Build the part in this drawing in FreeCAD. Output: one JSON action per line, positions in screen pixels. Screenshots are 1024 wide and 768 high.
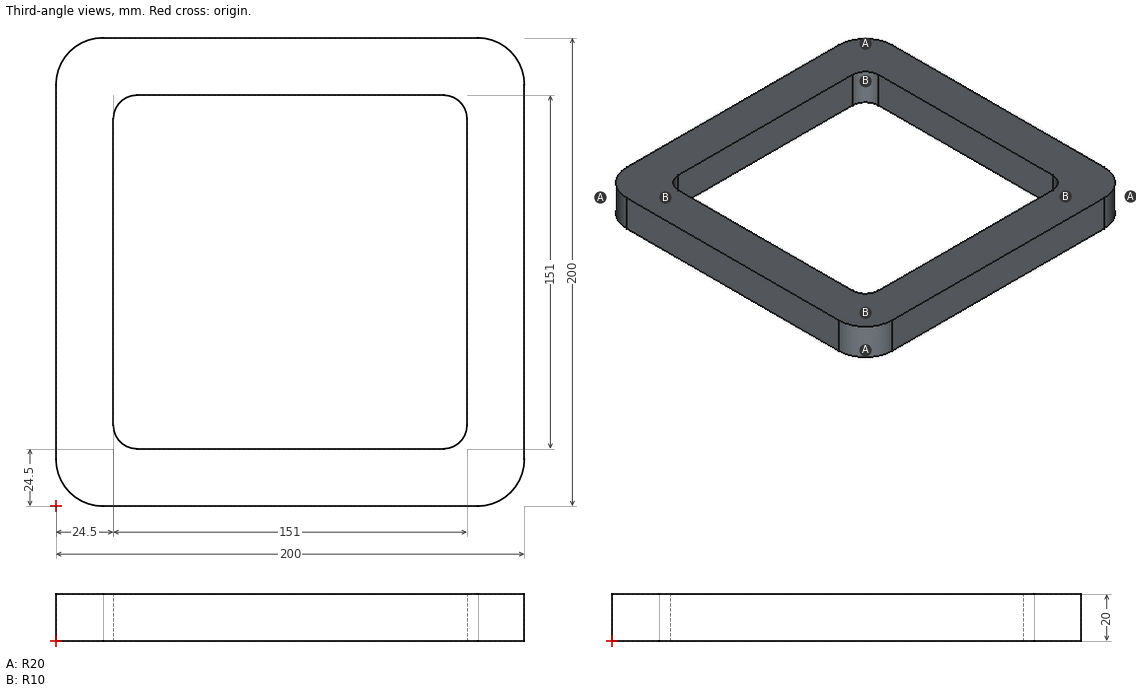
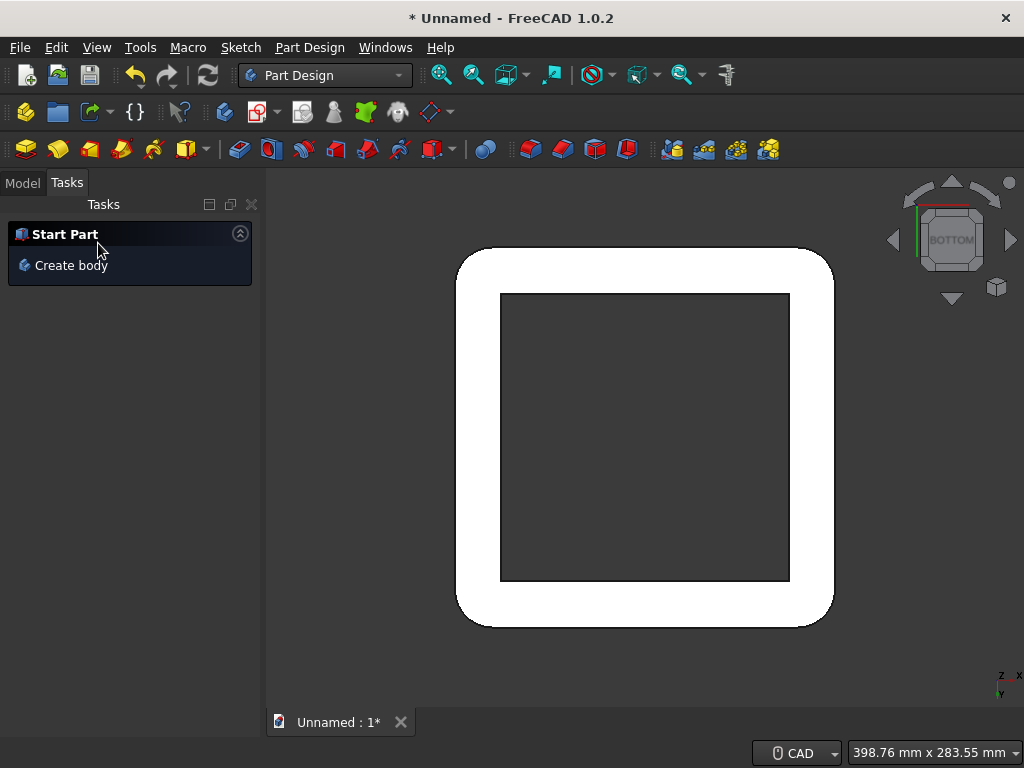
{"action": "key", "text": "4"}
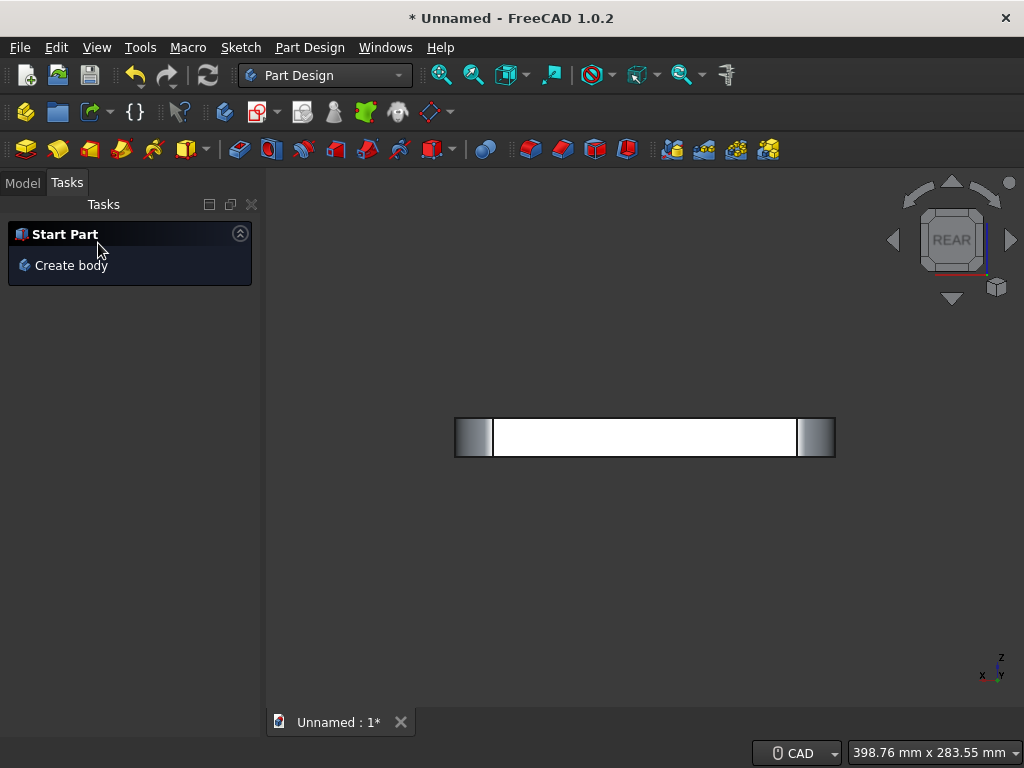
{"action": "key", "text": "6"}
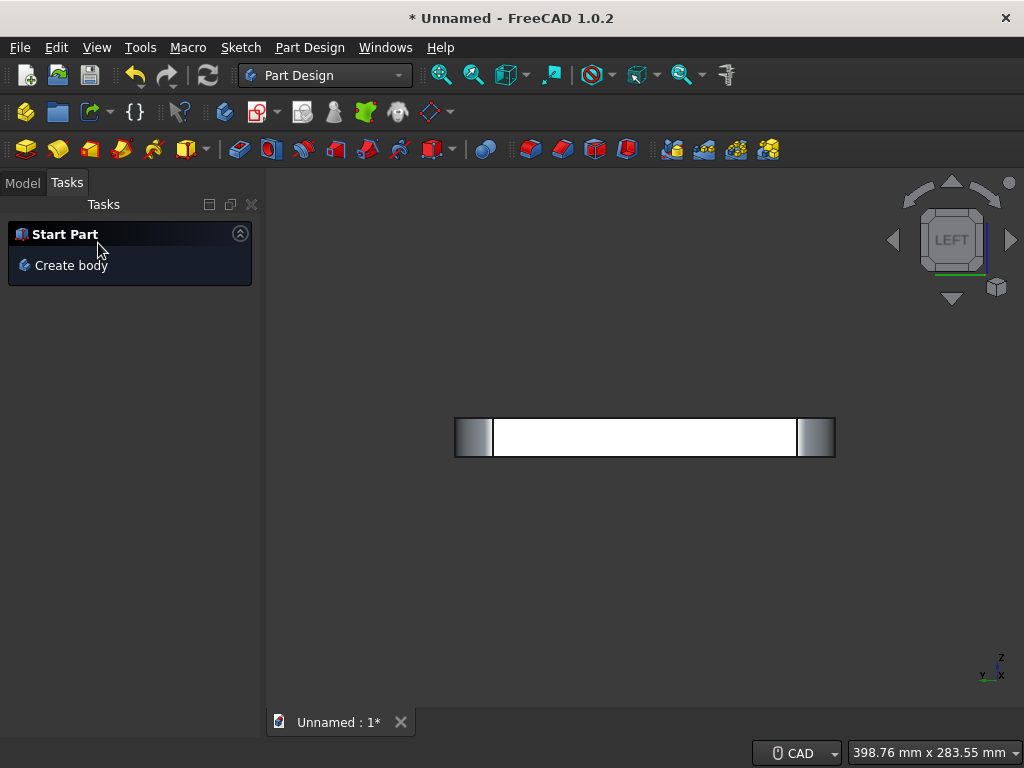
{"action": "key", "text": "v 3"}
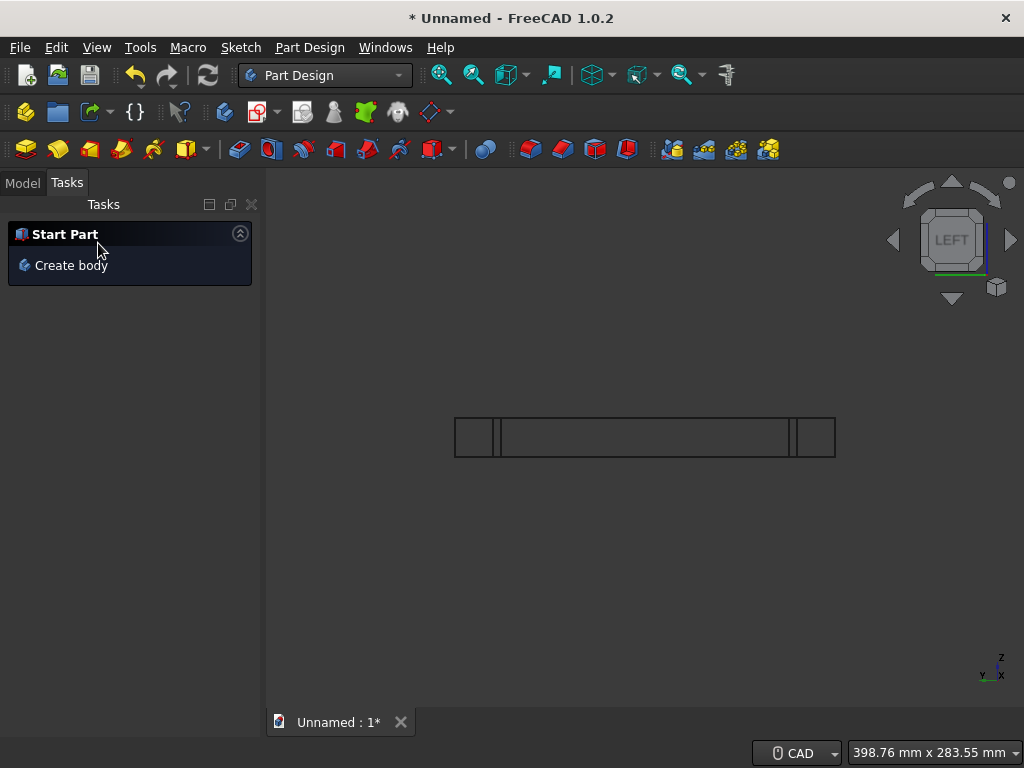
{"action": "key", "text": "0"}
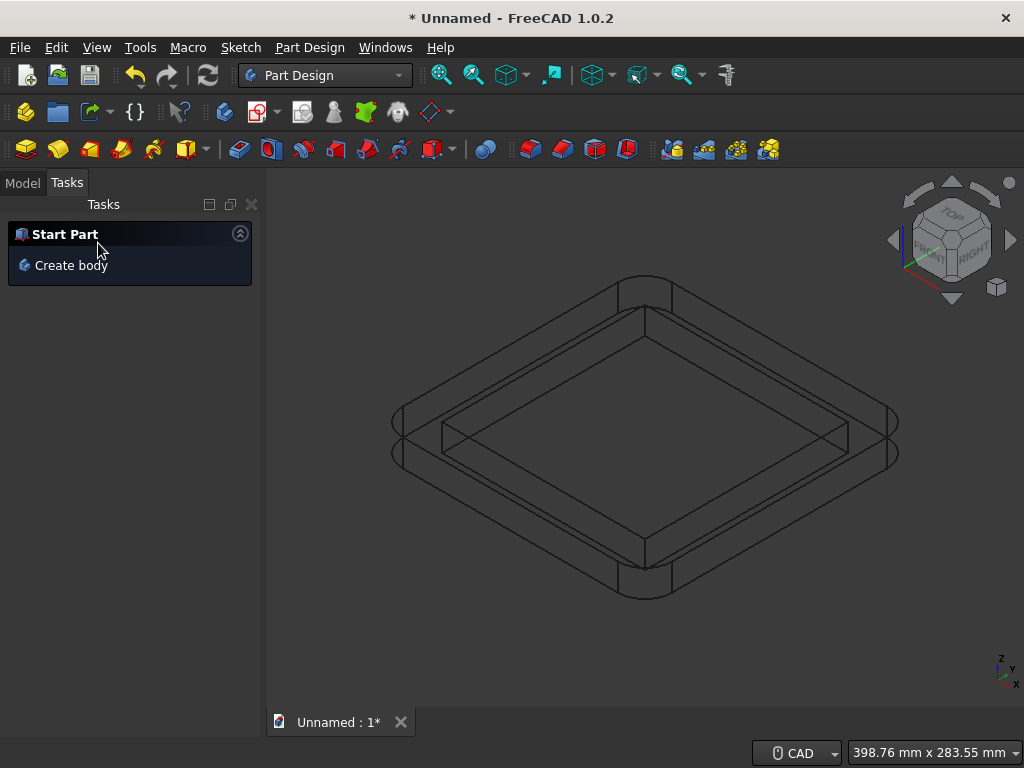
{"action": "left_click", "coordinate": [645, 319]}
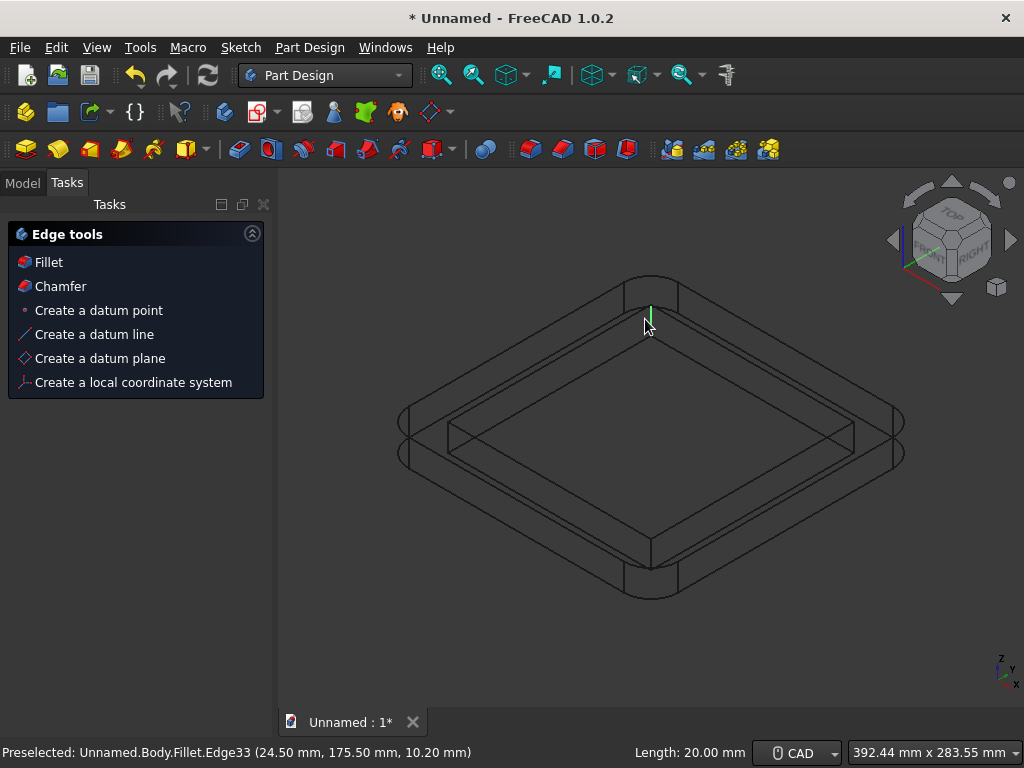
{"action": "left_click", "coordinate": [448, 436], "text": "ctrl"}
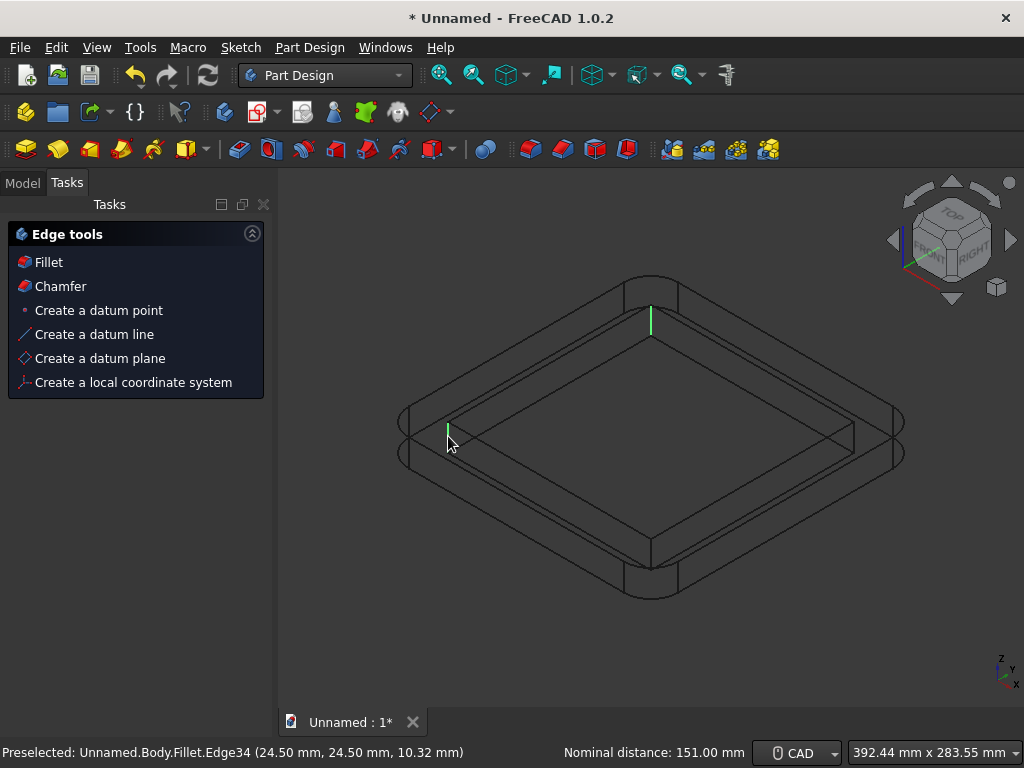
{"action": "left_click", "coordinate": [651, 554], "text": "ctrl"}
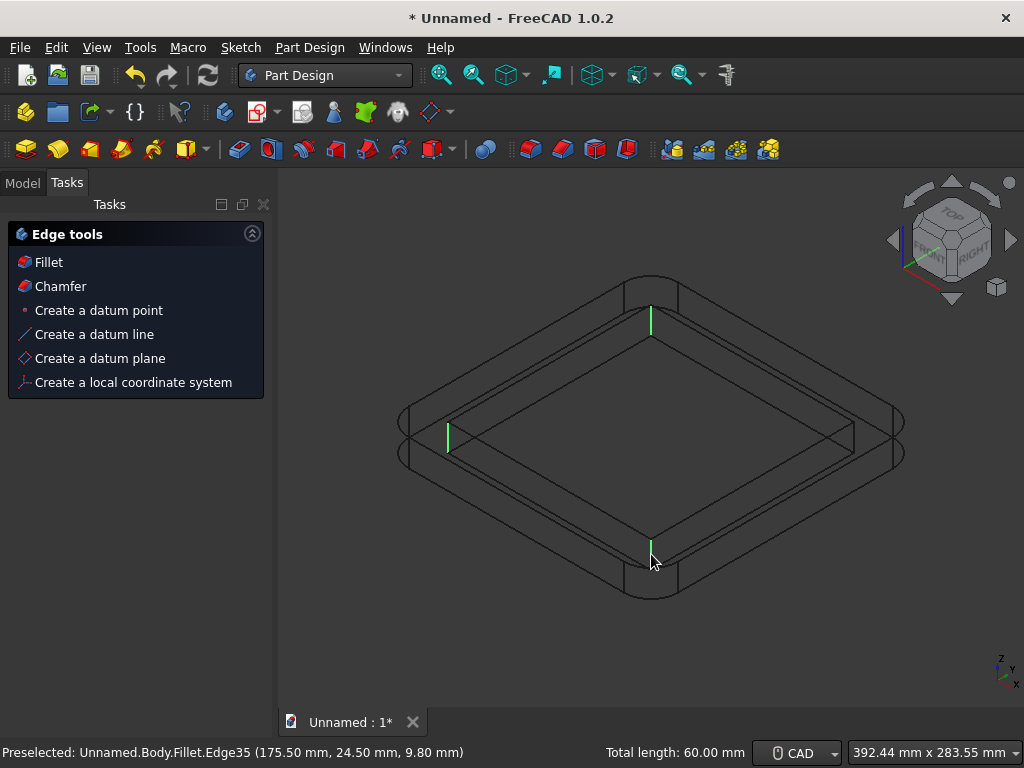
{"action": "left_click", "coordinate": [854, 436], "text": "ctrl"}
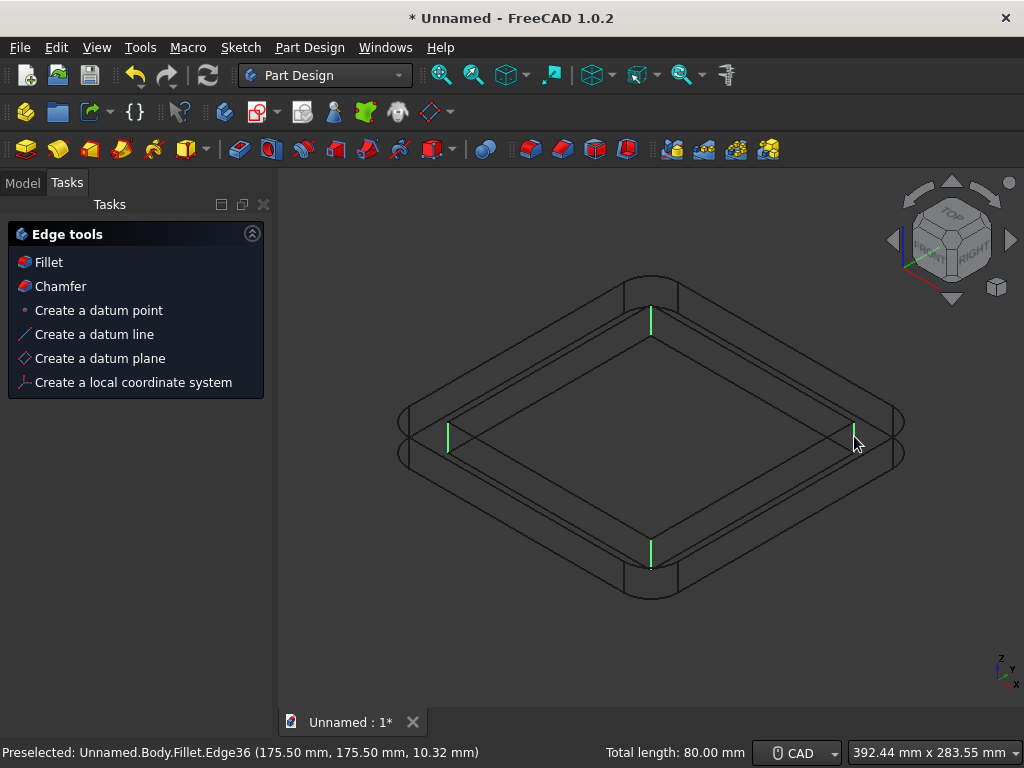
{"action": "key", "text": "v 1"}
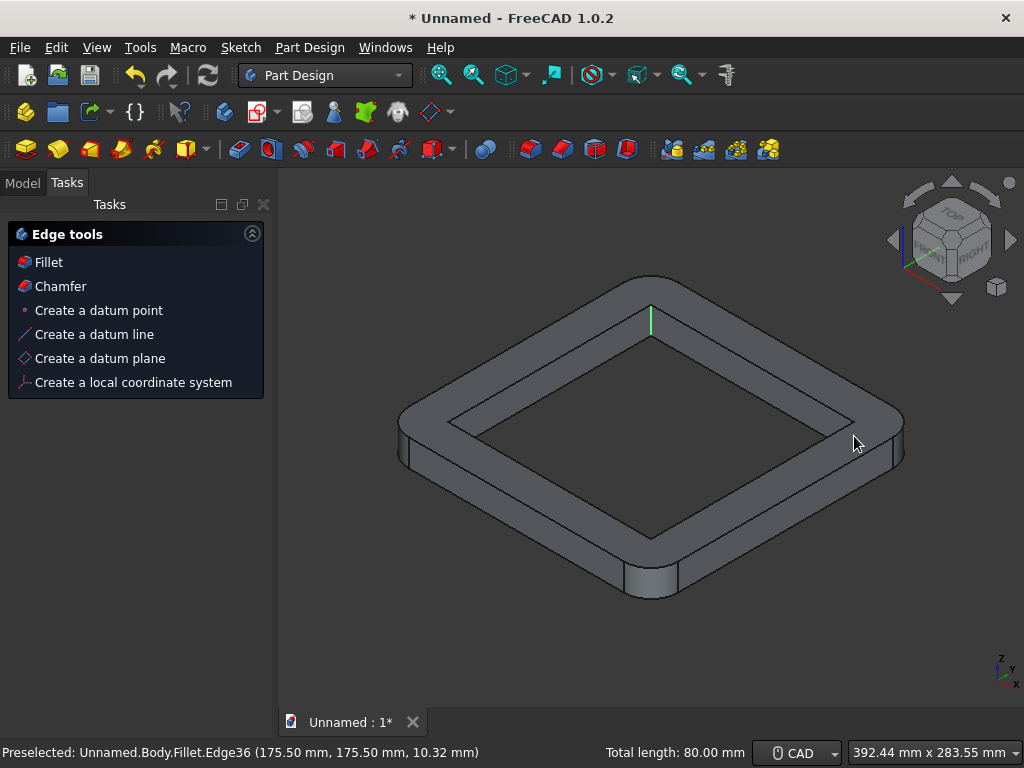
{"action": "left_click", "coordinate": [532, 150]}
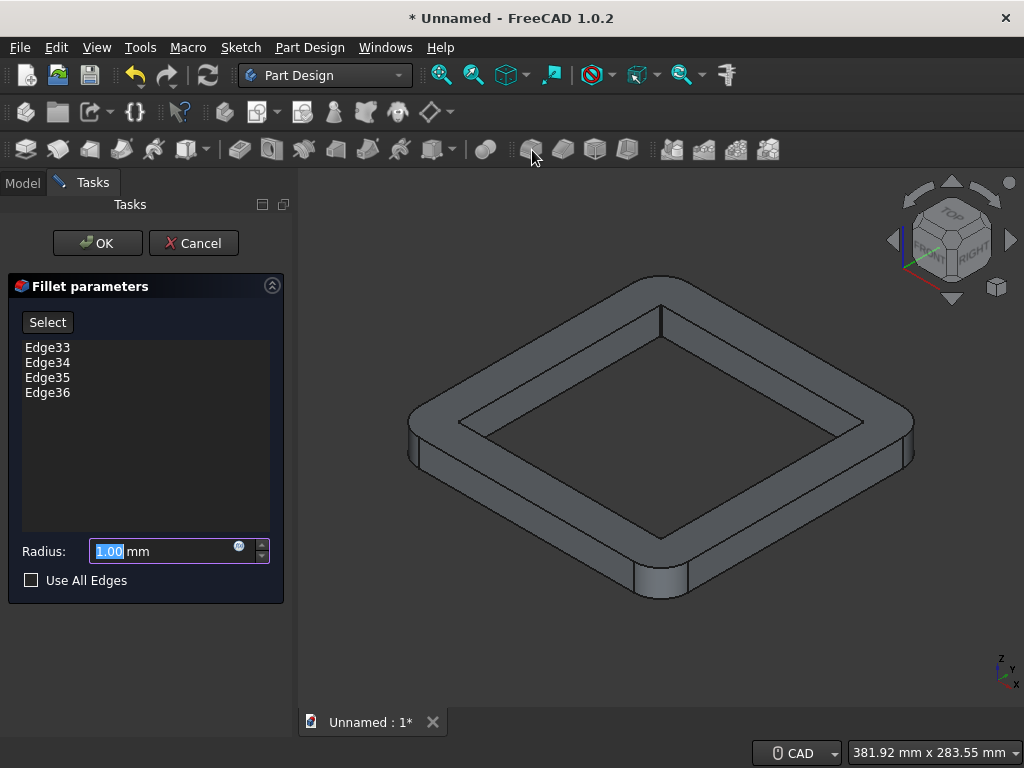
{"action": "type", "text": "10"}
{"action": "key", "text": "Tab"}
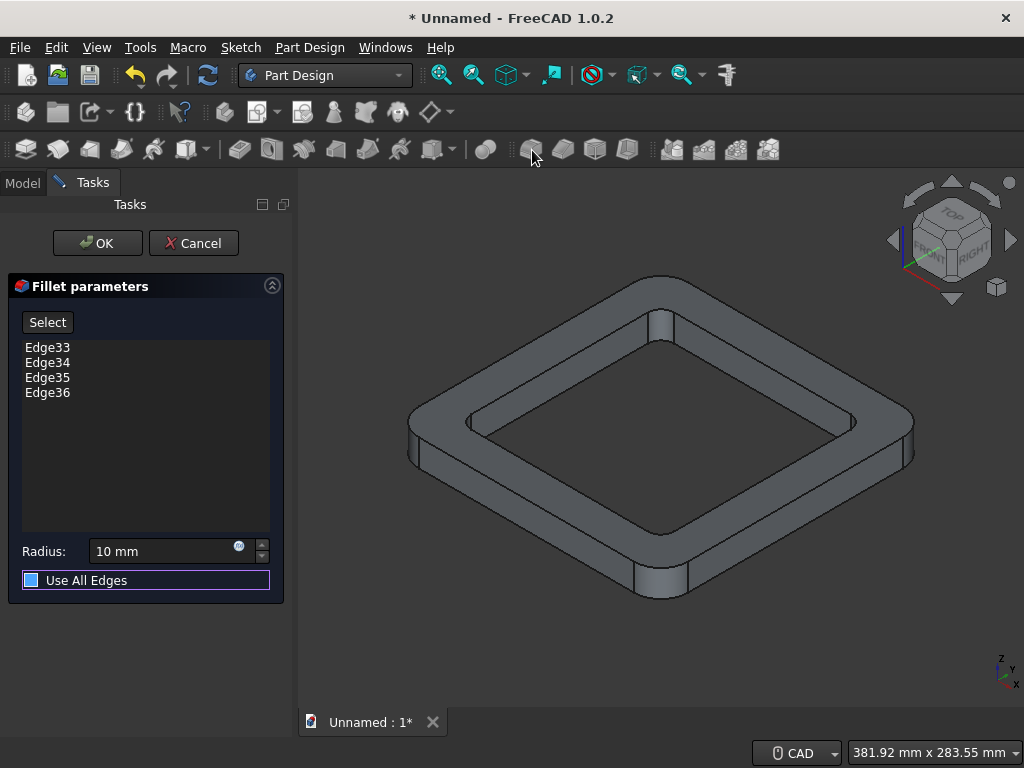
{"action": "left_click", "coordinate": [98, 243]}